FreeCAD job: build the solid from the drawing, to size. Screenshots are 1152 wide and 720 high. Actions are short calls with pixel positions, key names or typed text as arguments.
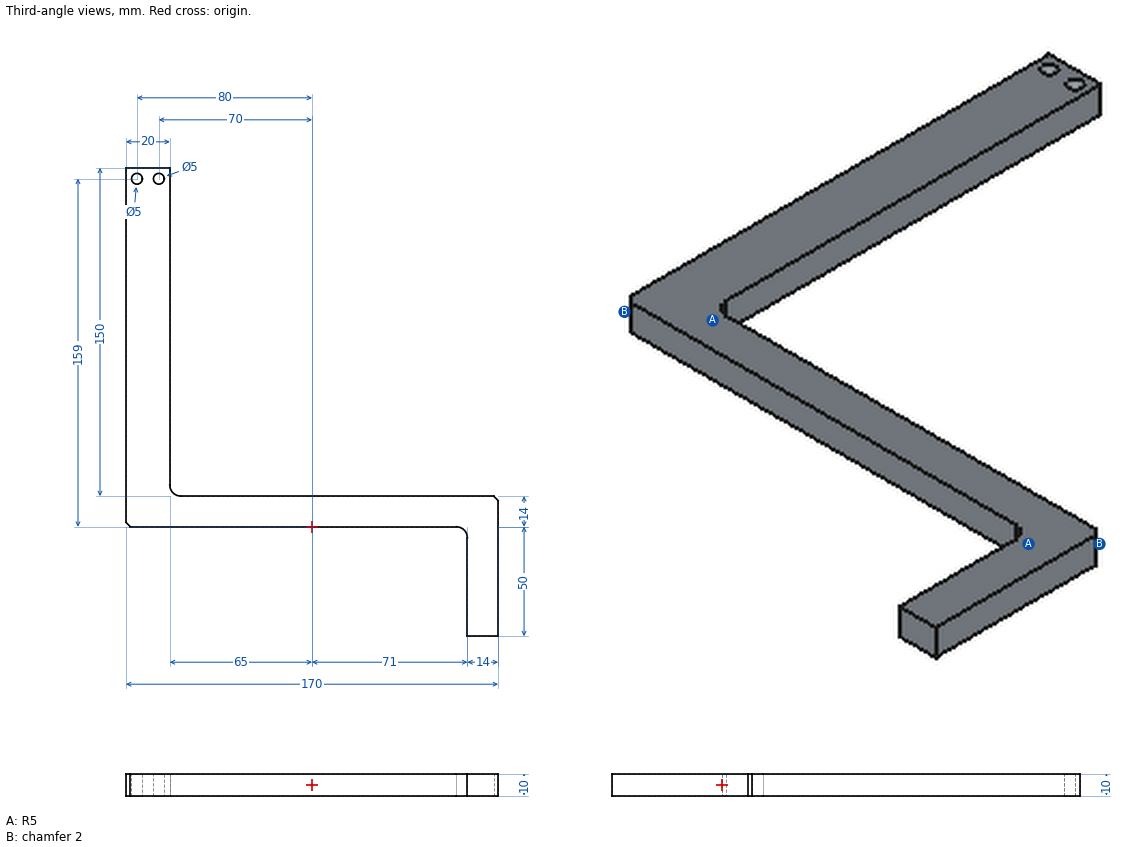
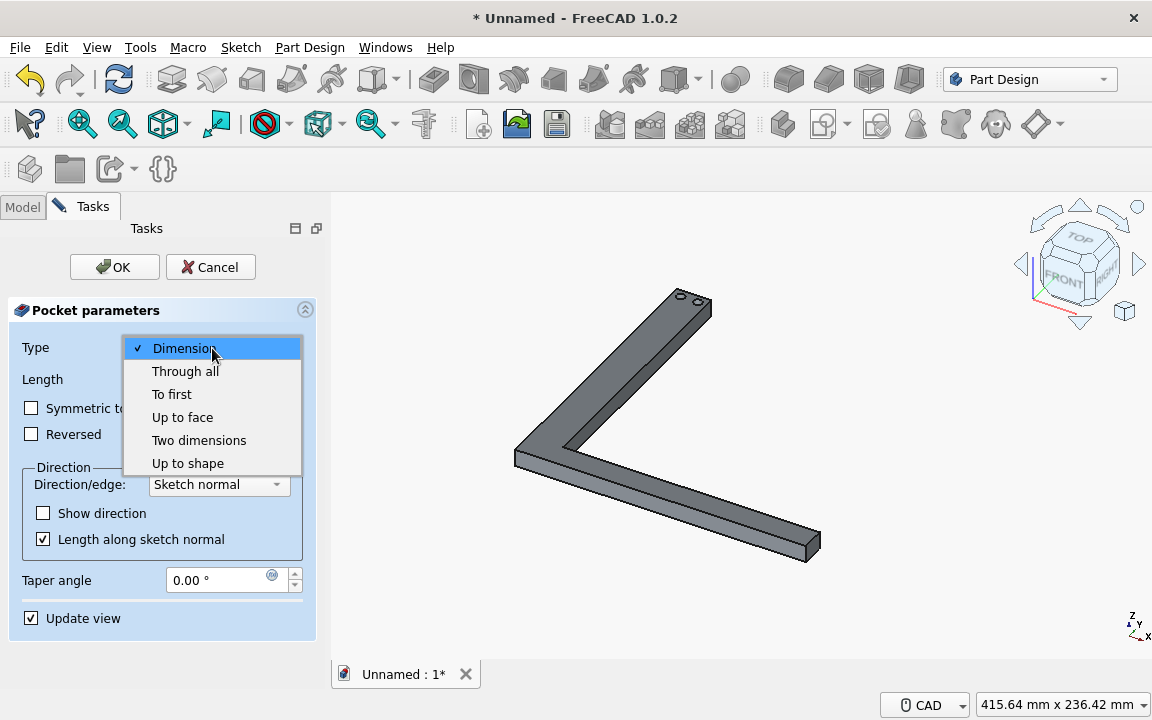
click(212, 394)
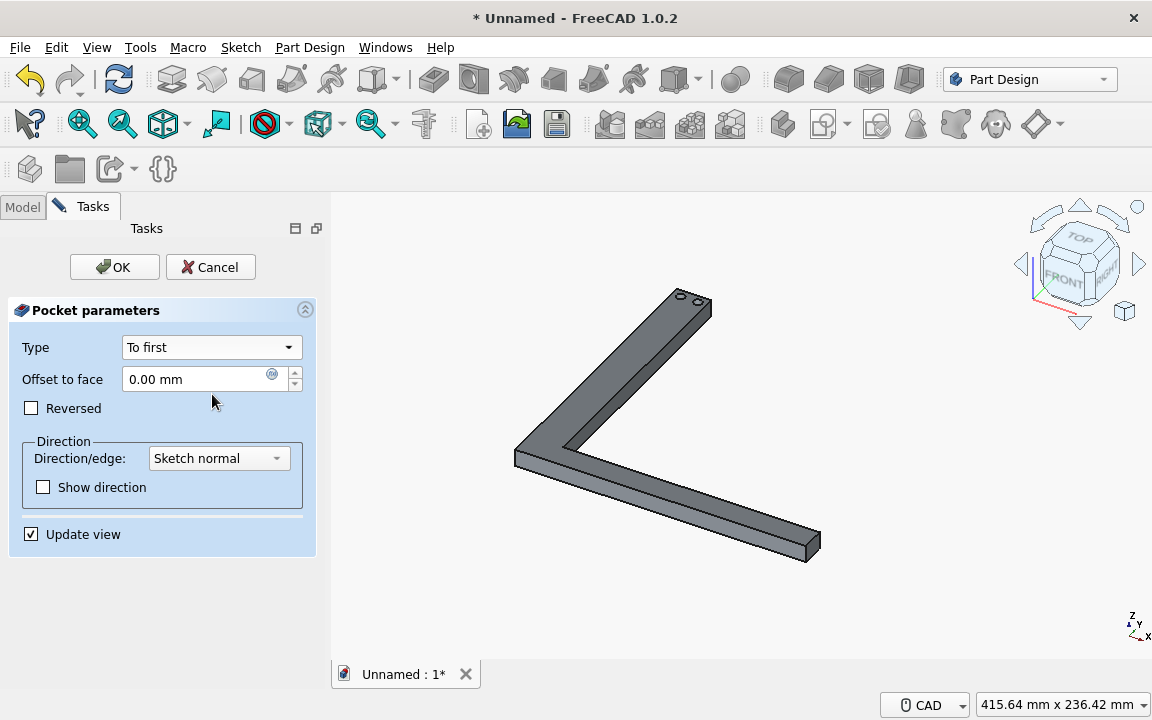
click(115, 267)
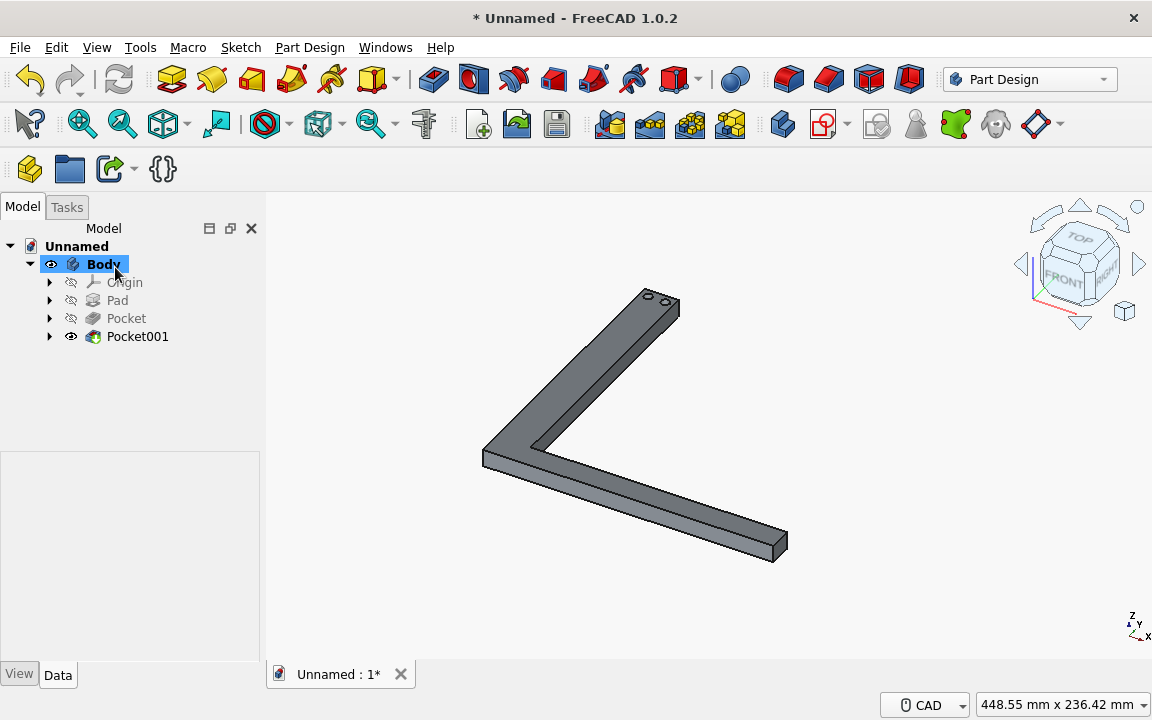
click(515, 444)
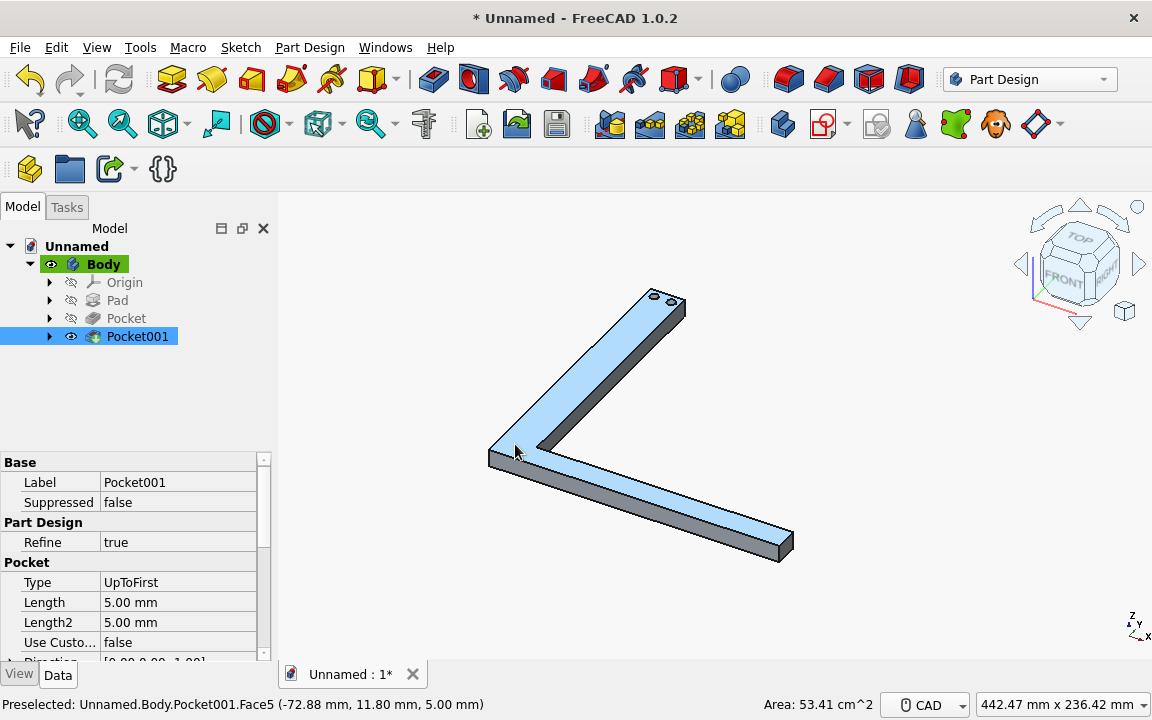
click(824, 124)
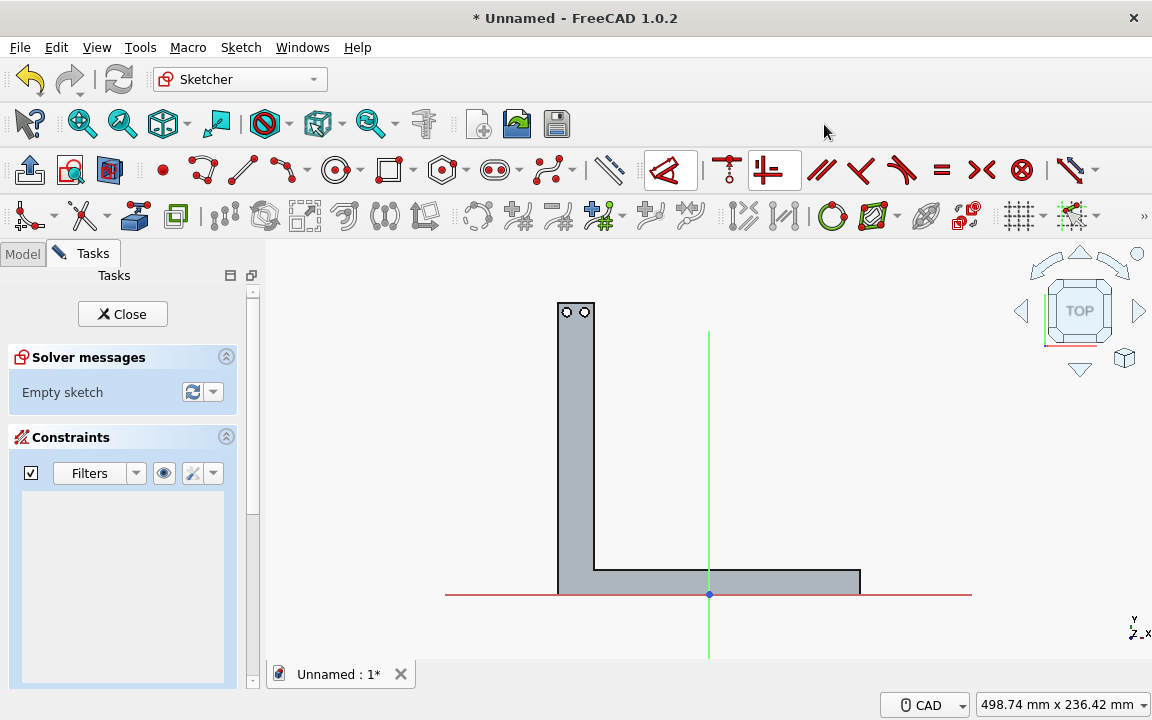
scroll(640, 449, down, 5)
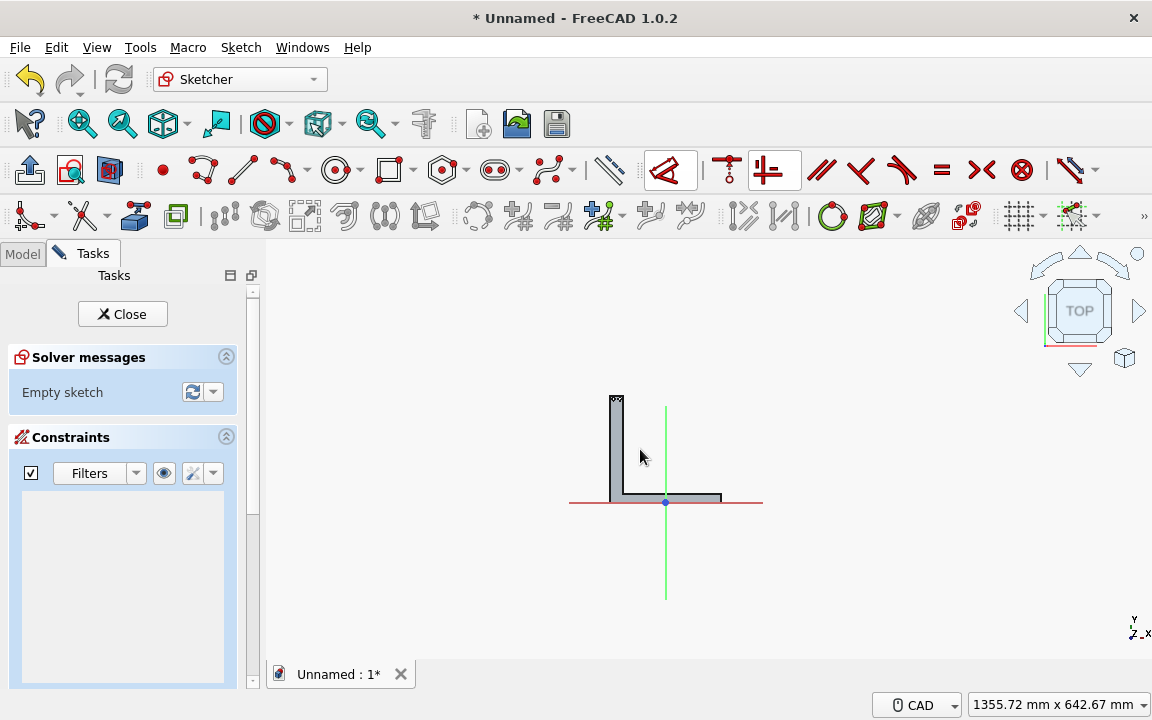
scroll(702, 530, up, 10)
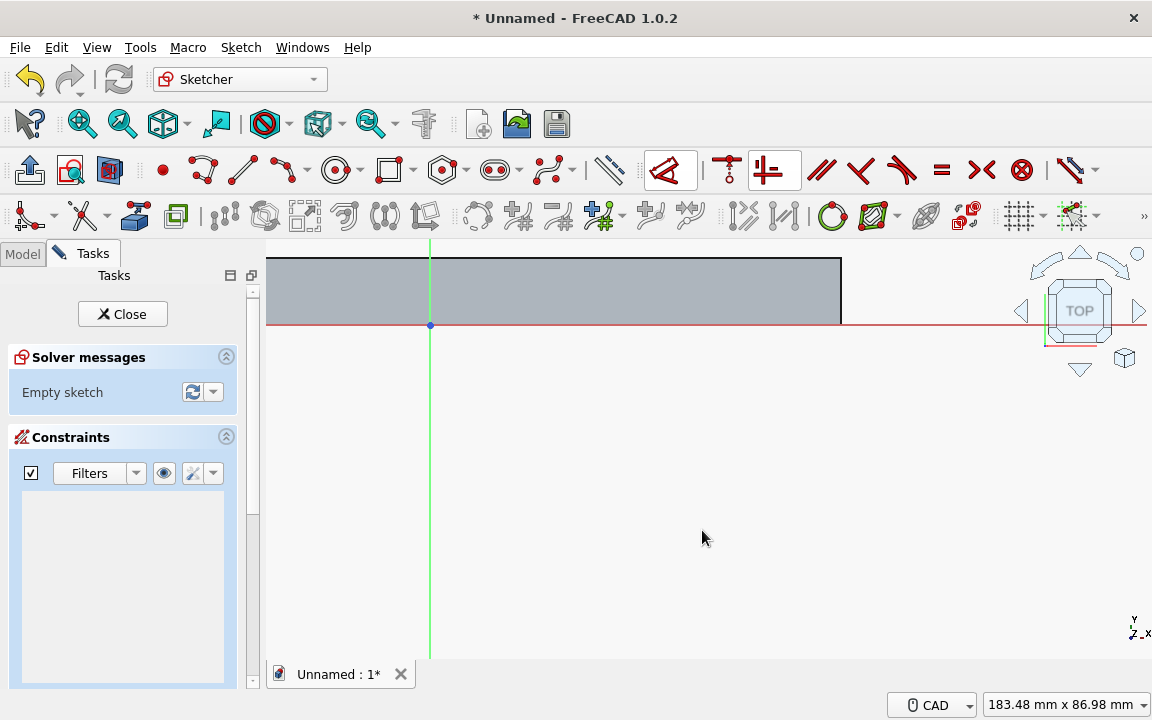
key(g)
key(r)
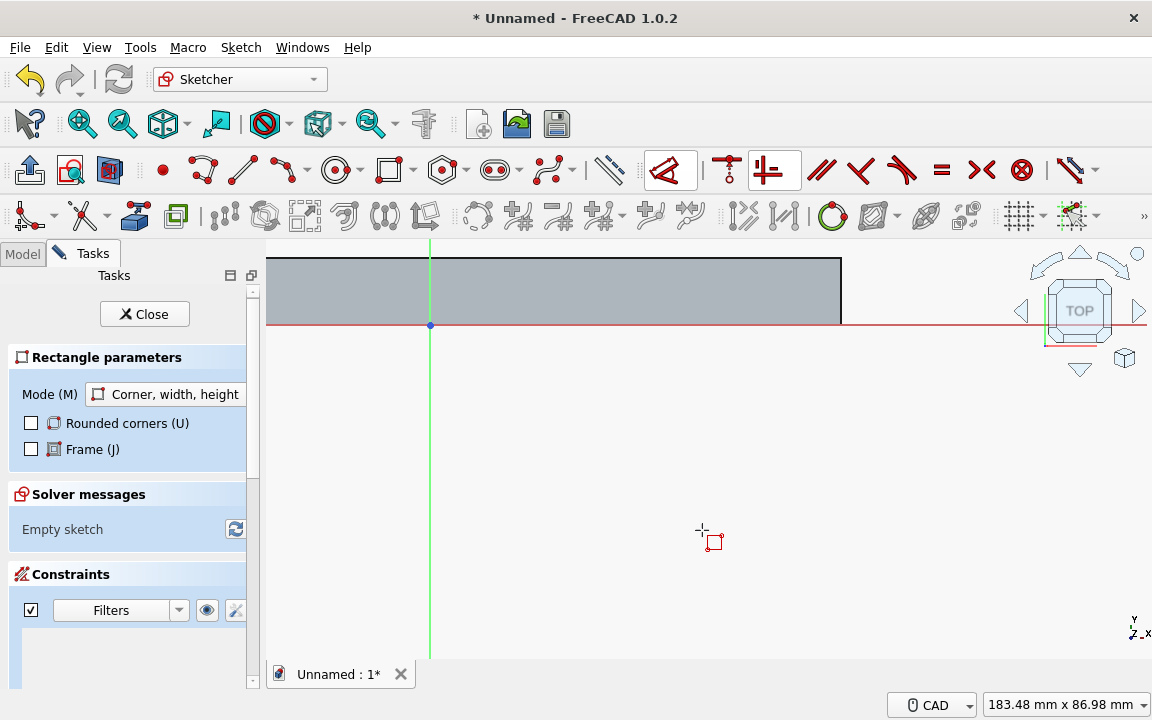
click(773, 325)
move(841, 567)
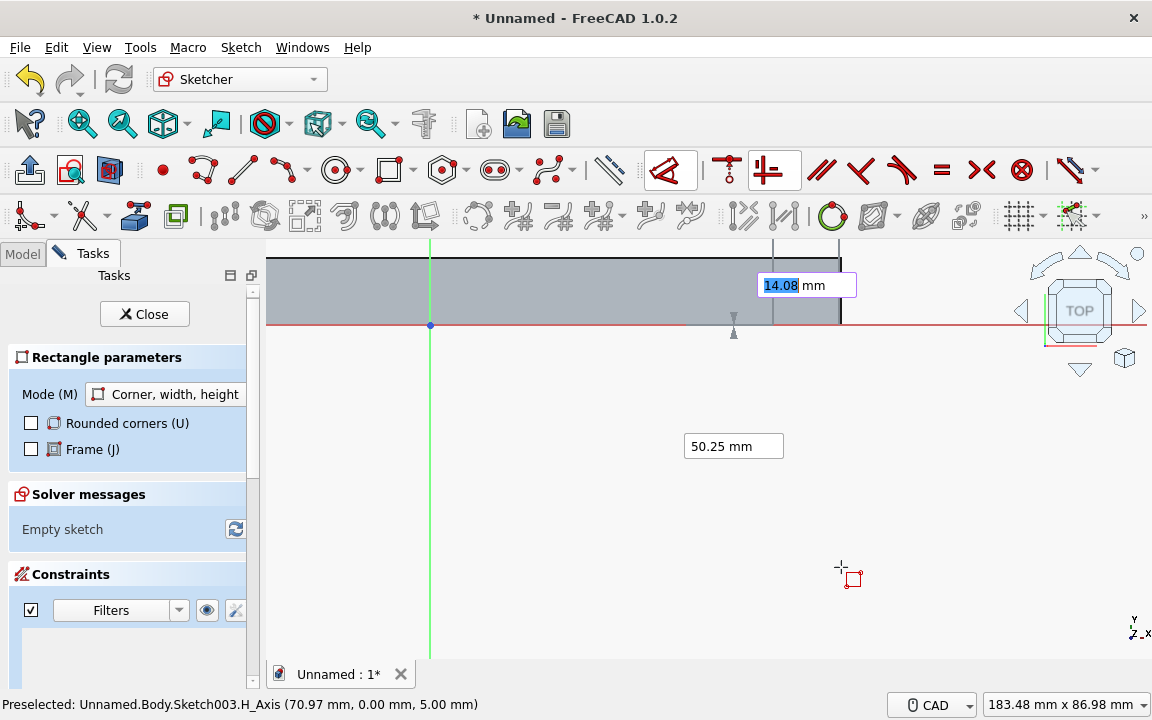
text(14)
key(Tab)
text(50)
key(Return)
key(Escape)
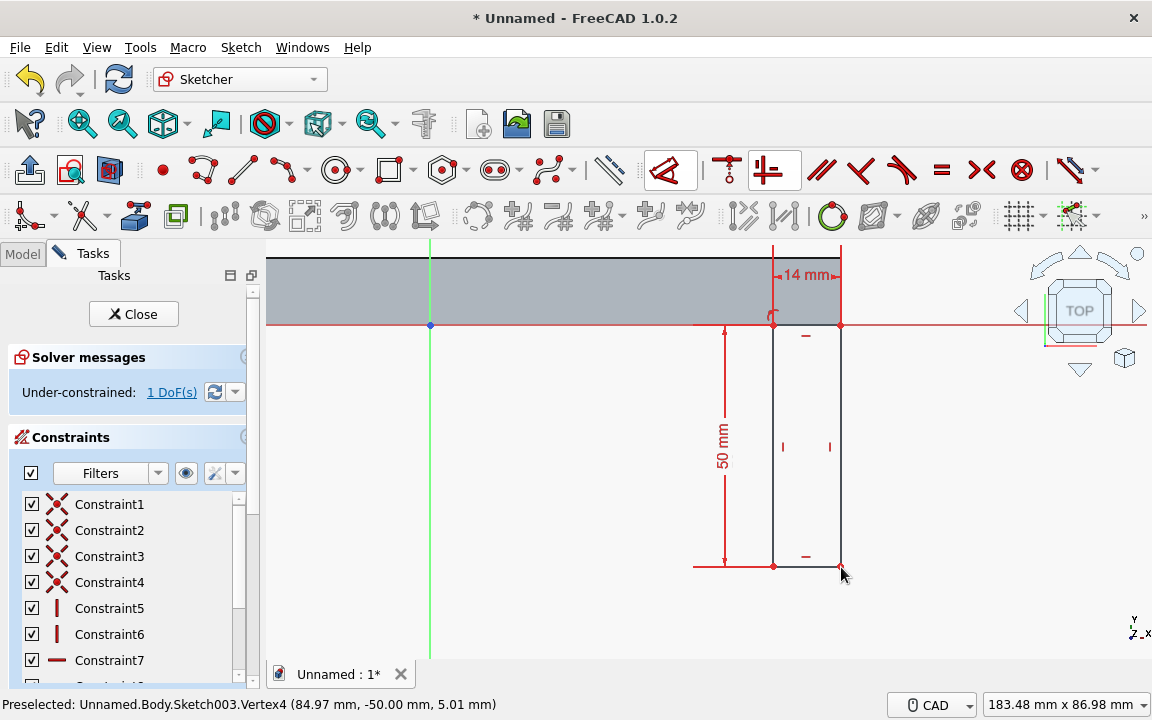
key(d)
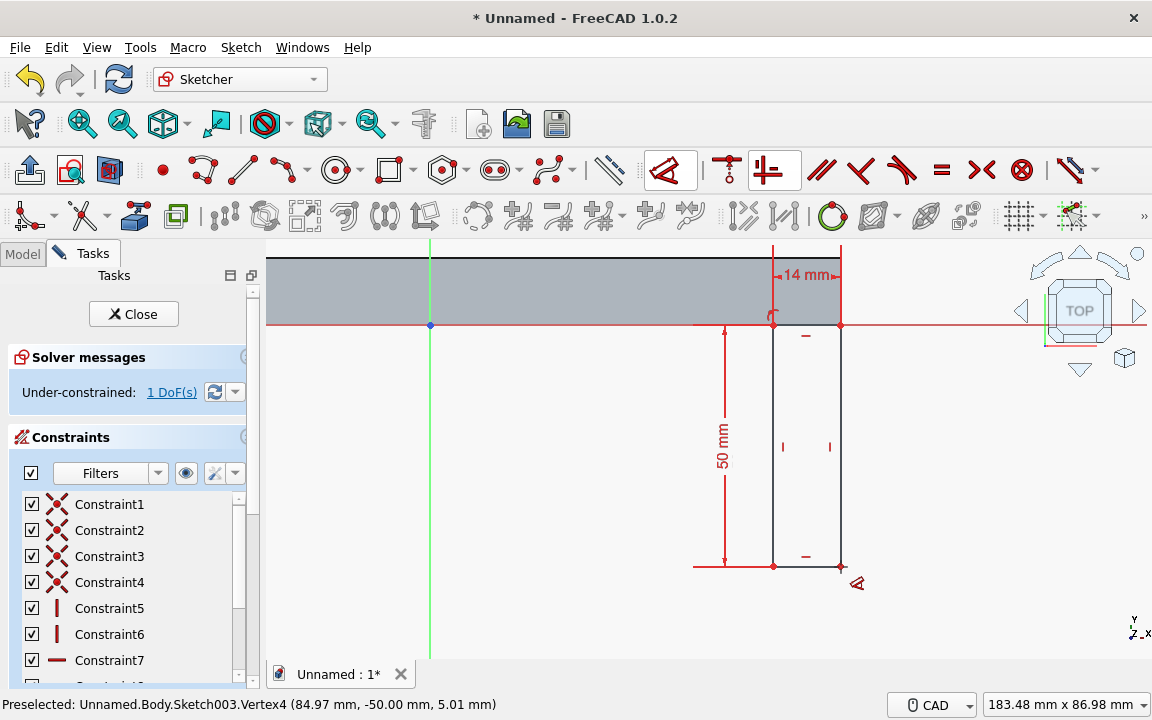
click(773, 325)
click(602, 291)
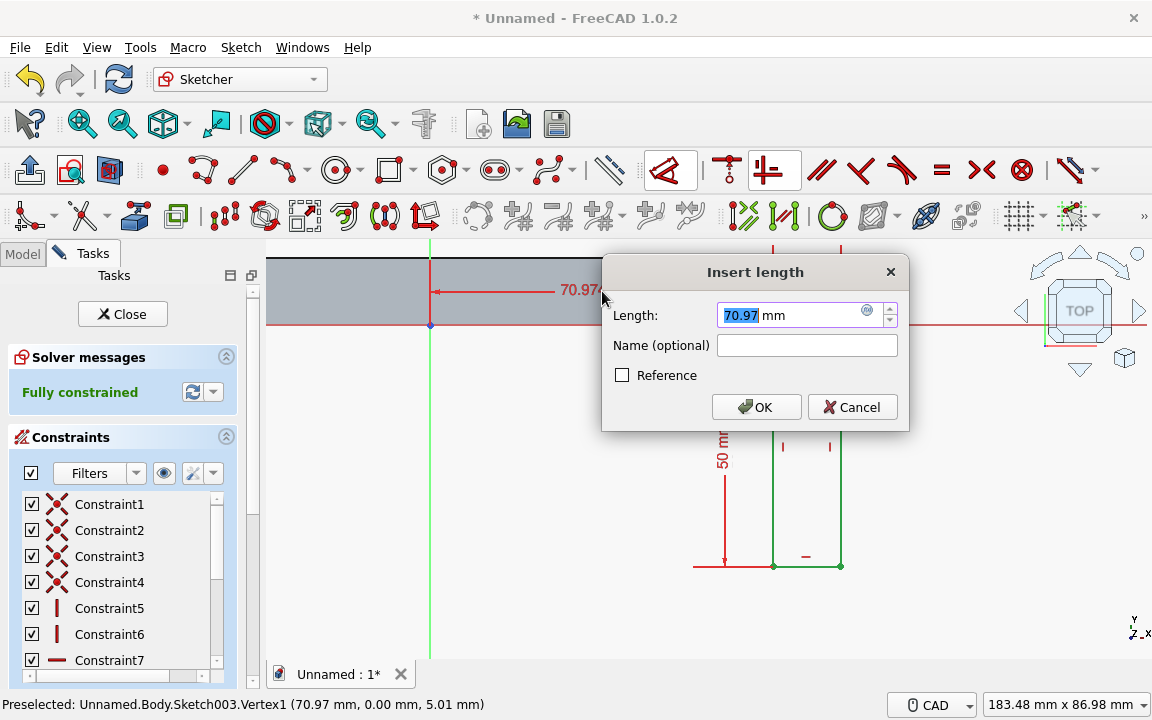
text(71)
key(Return)
key(Escape)